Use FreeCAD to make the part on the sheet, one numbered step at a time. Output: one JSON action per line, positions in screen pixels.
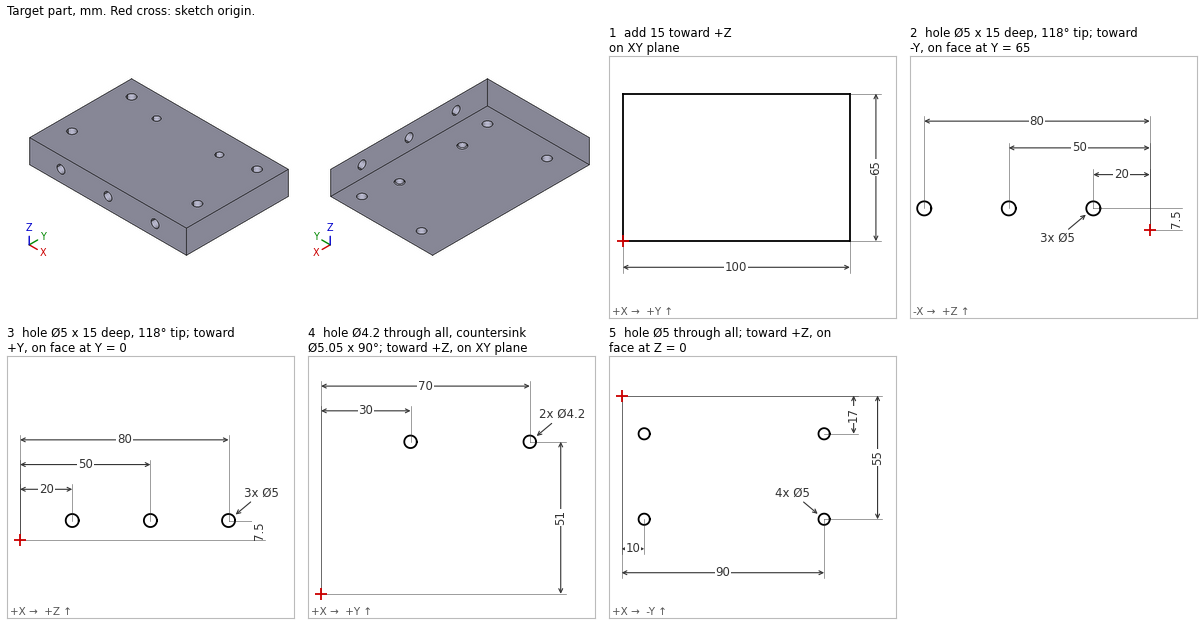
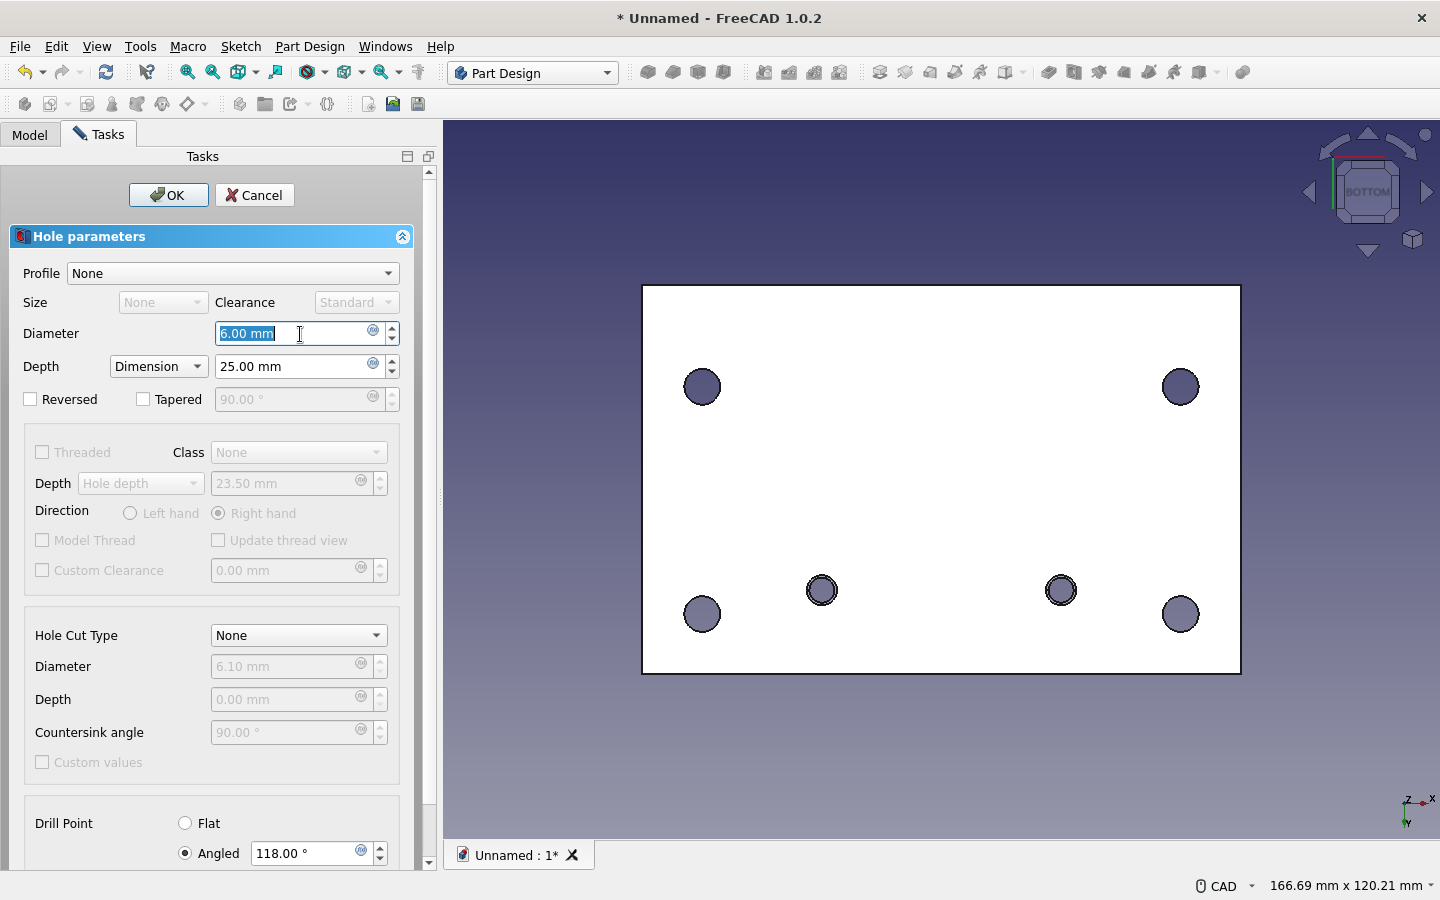
{"action": "type", "text": "5"}
{"action": "key", "text": "Tab"}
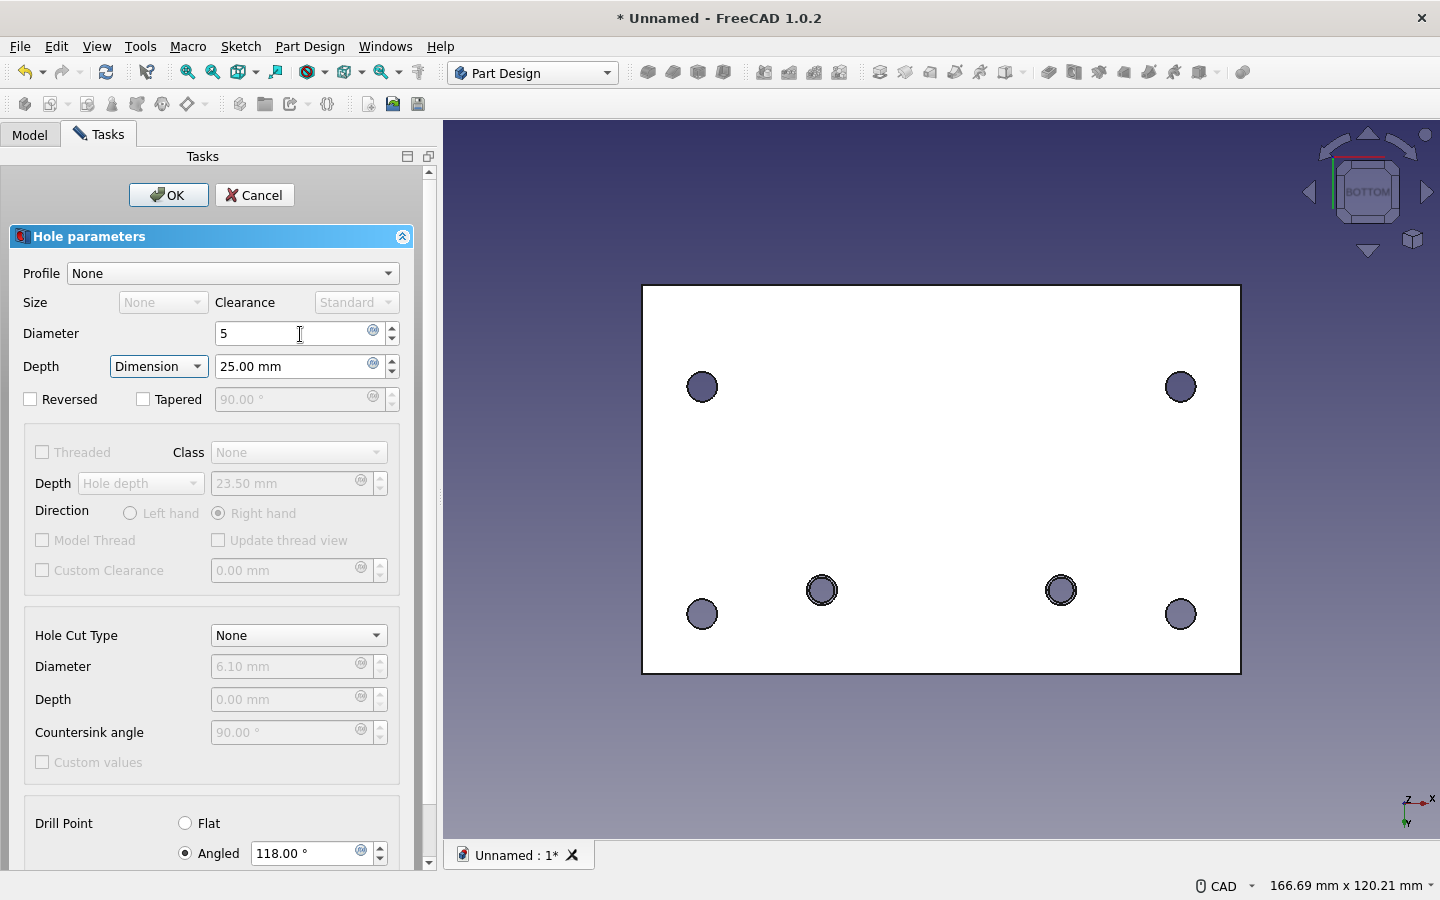
{"action": "left_click", "coordinate": [160, 366]}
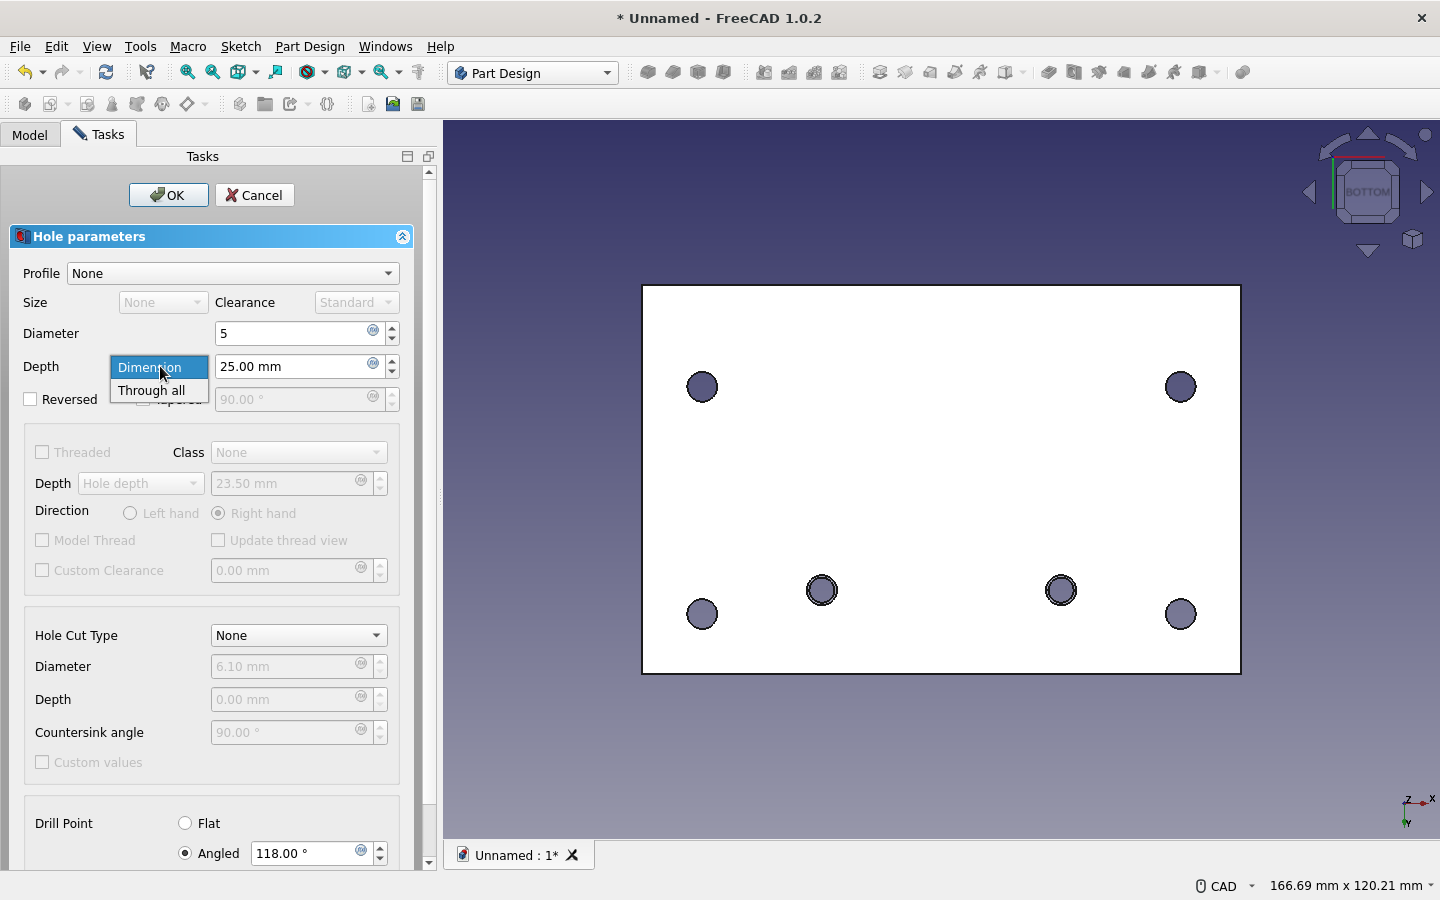
{"action": "left_click", "coordinate": [158, 390]}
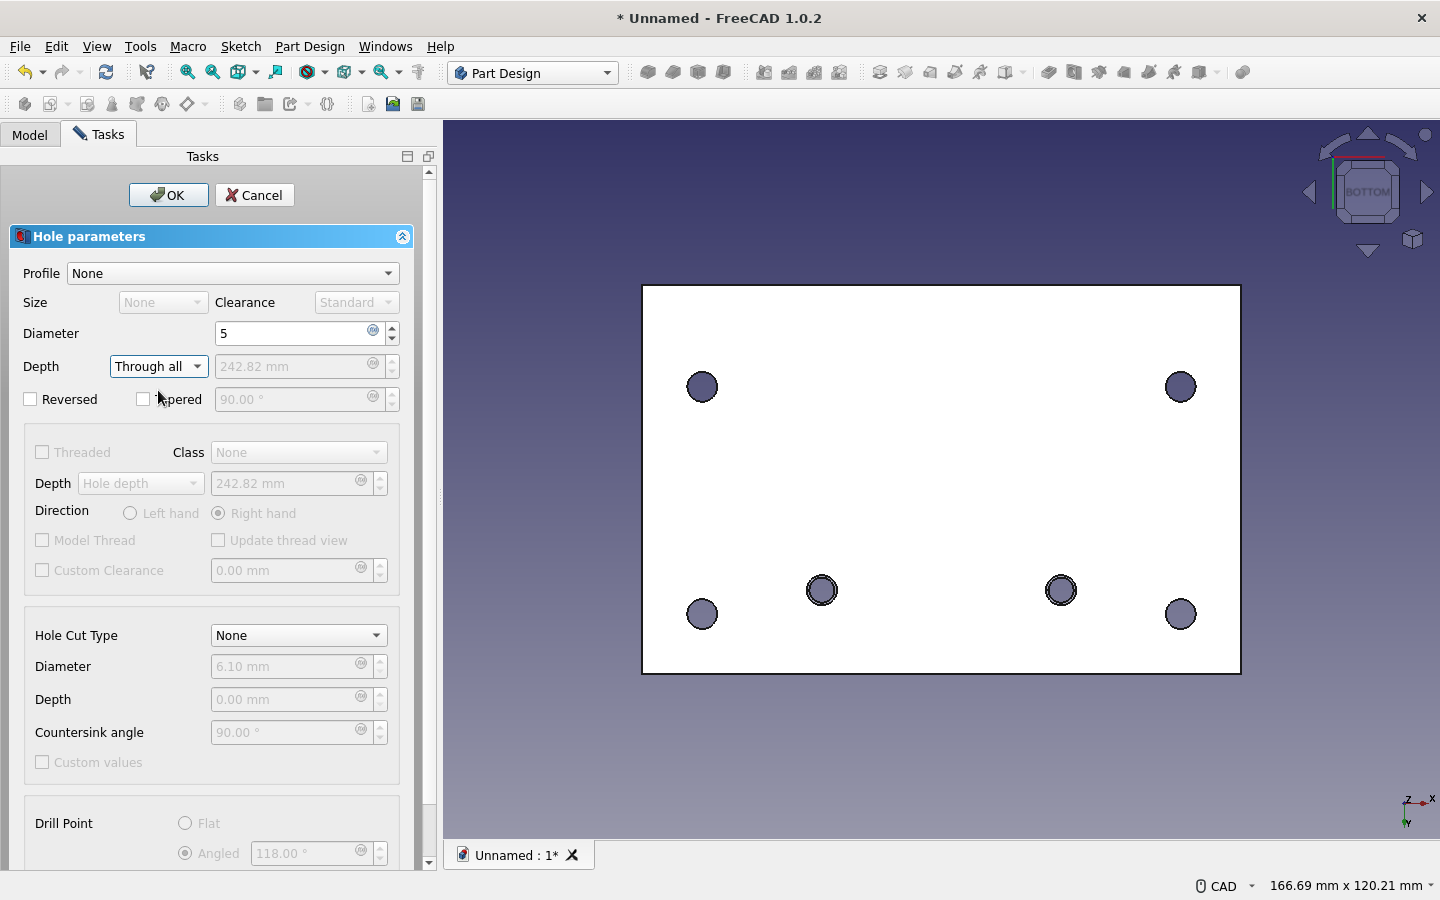
{"action": "left_click", "coordinate": [169, 195]}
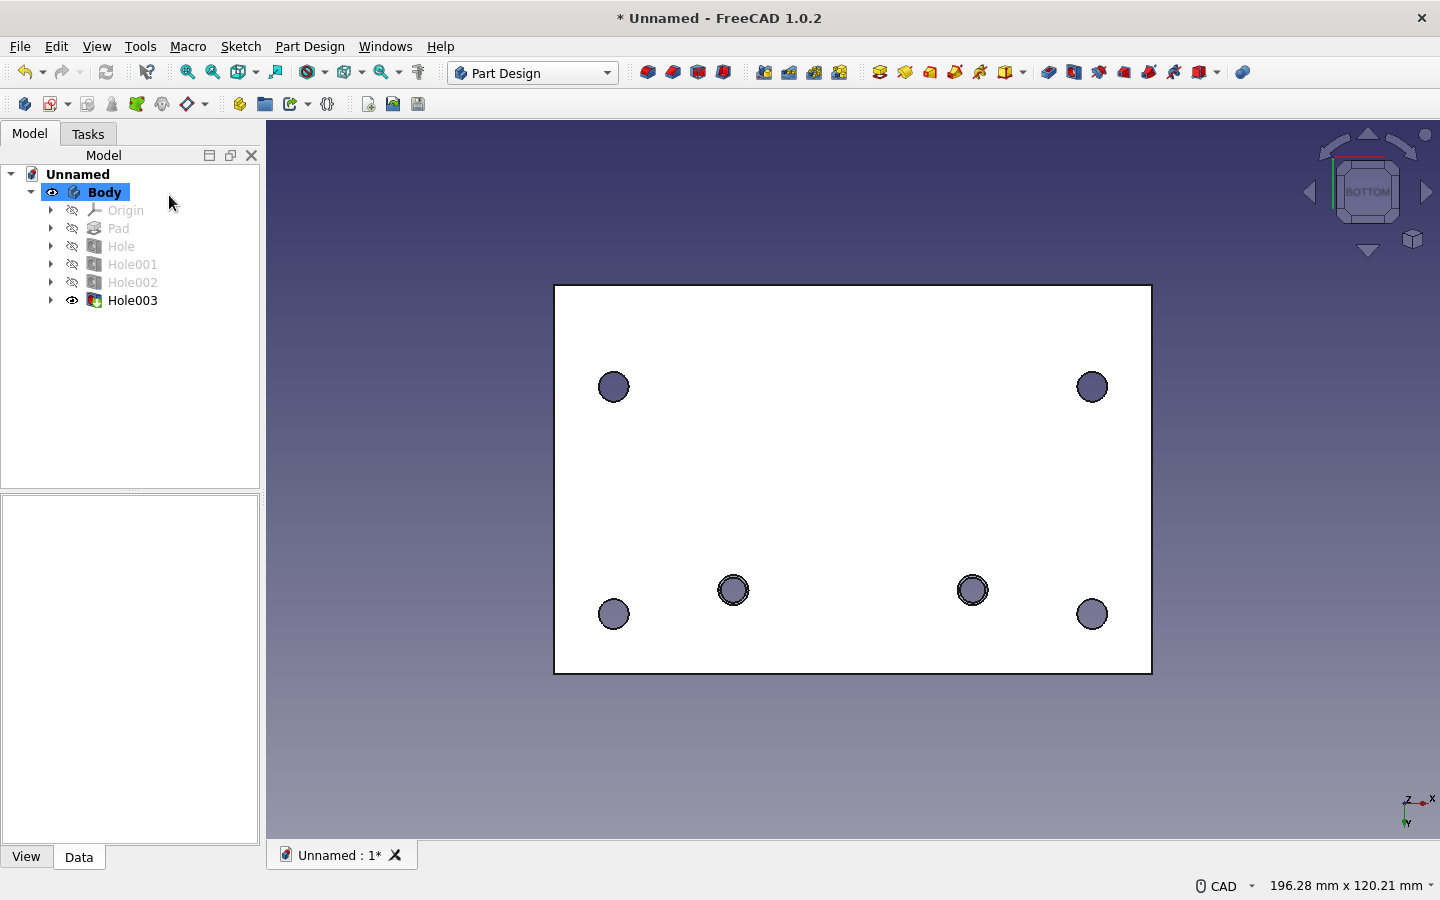
{"action": "key", "text": "0"}